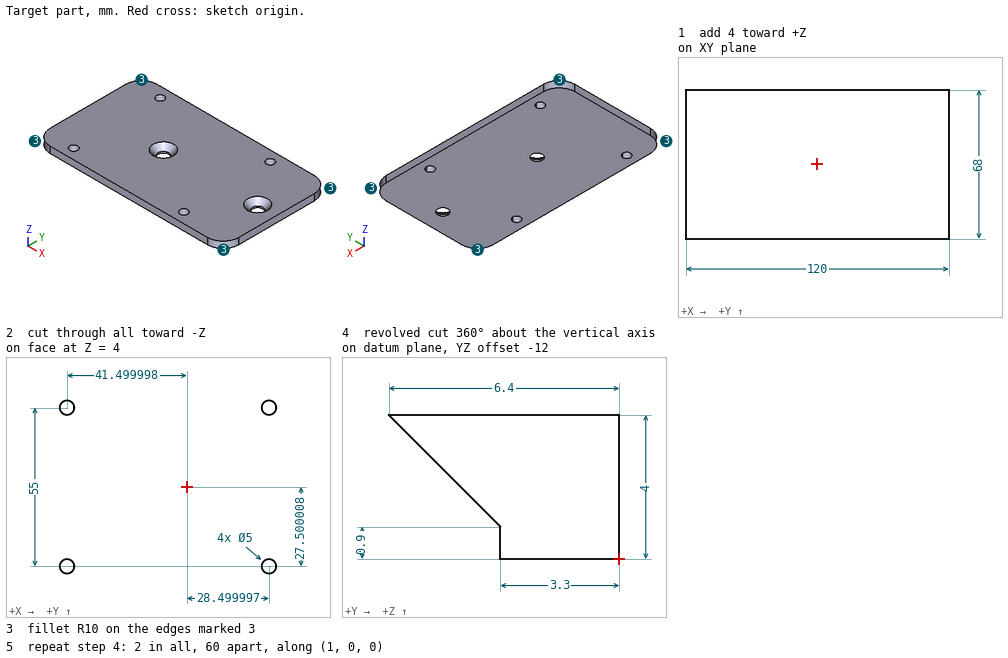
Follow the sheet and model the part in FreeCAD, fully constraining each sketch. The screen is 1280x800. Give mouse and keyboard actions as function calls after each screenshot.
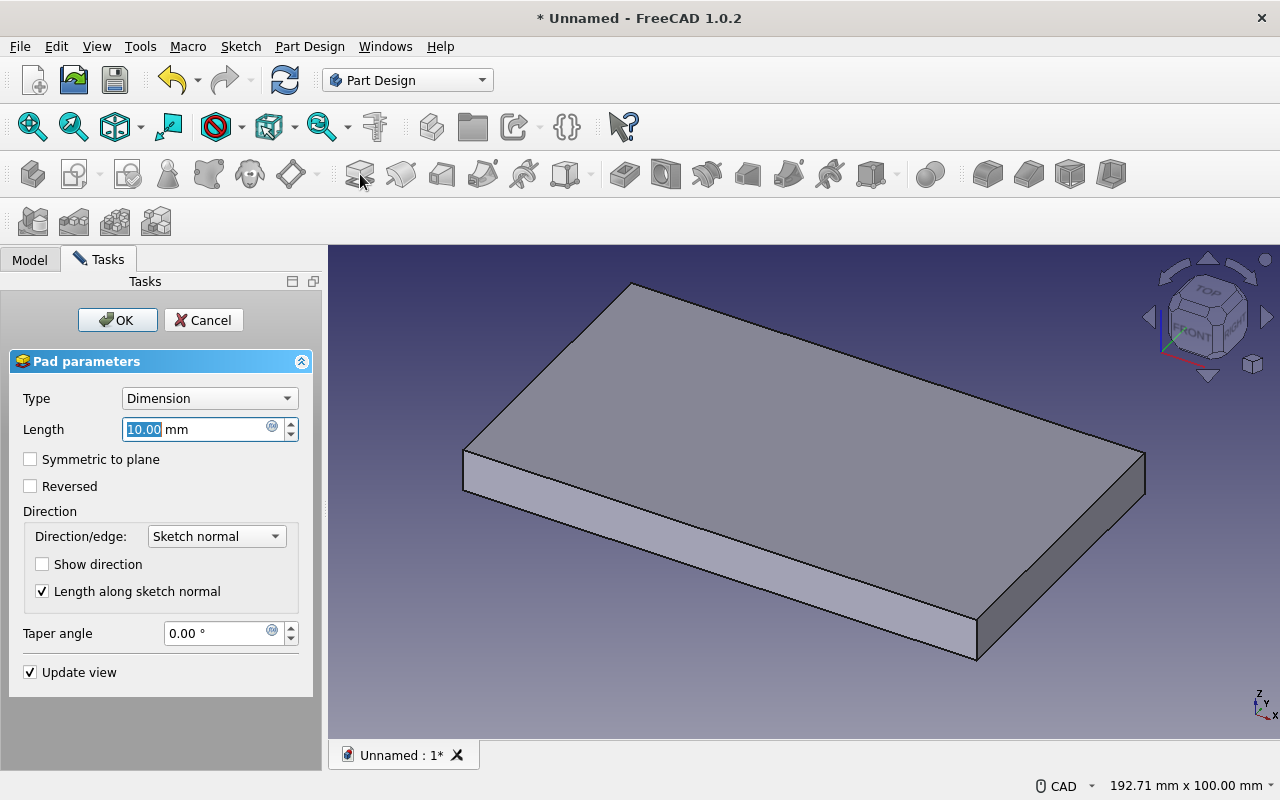
text(4)
key(Tab)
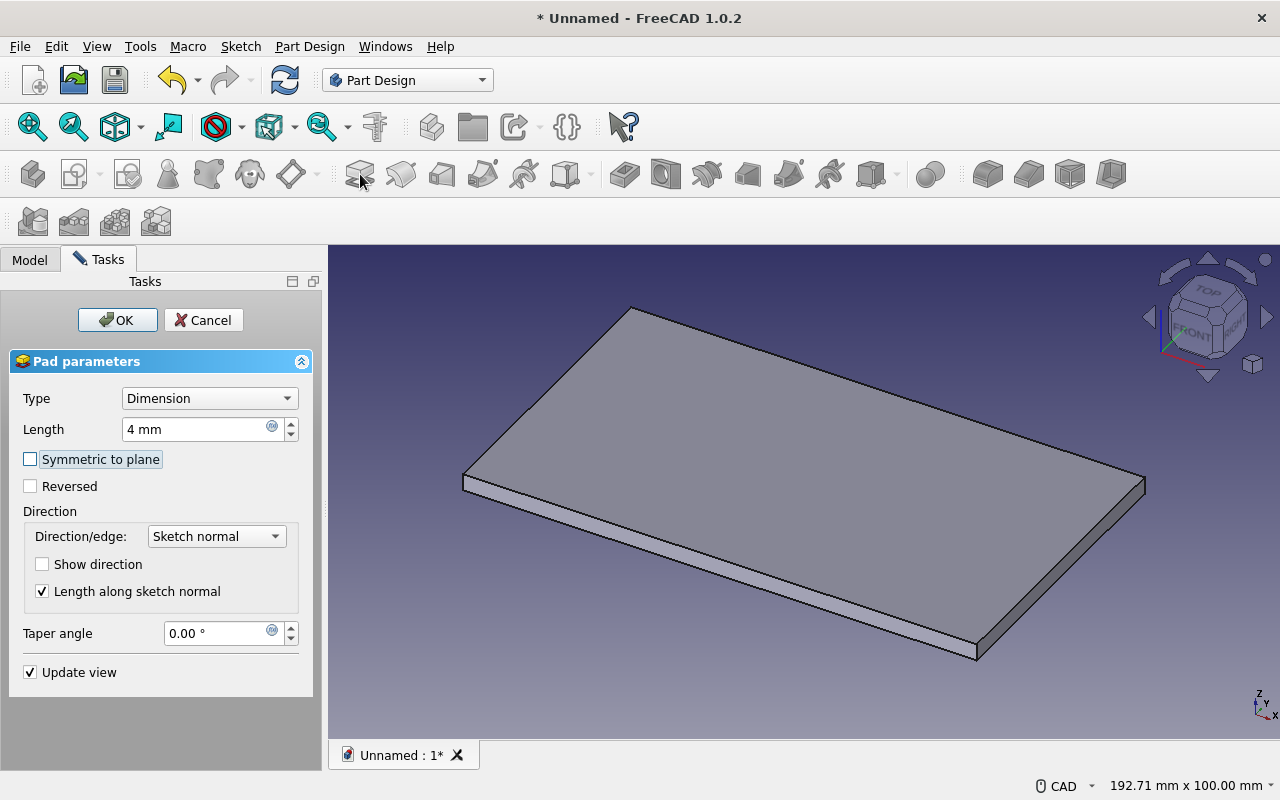
click(118, 320)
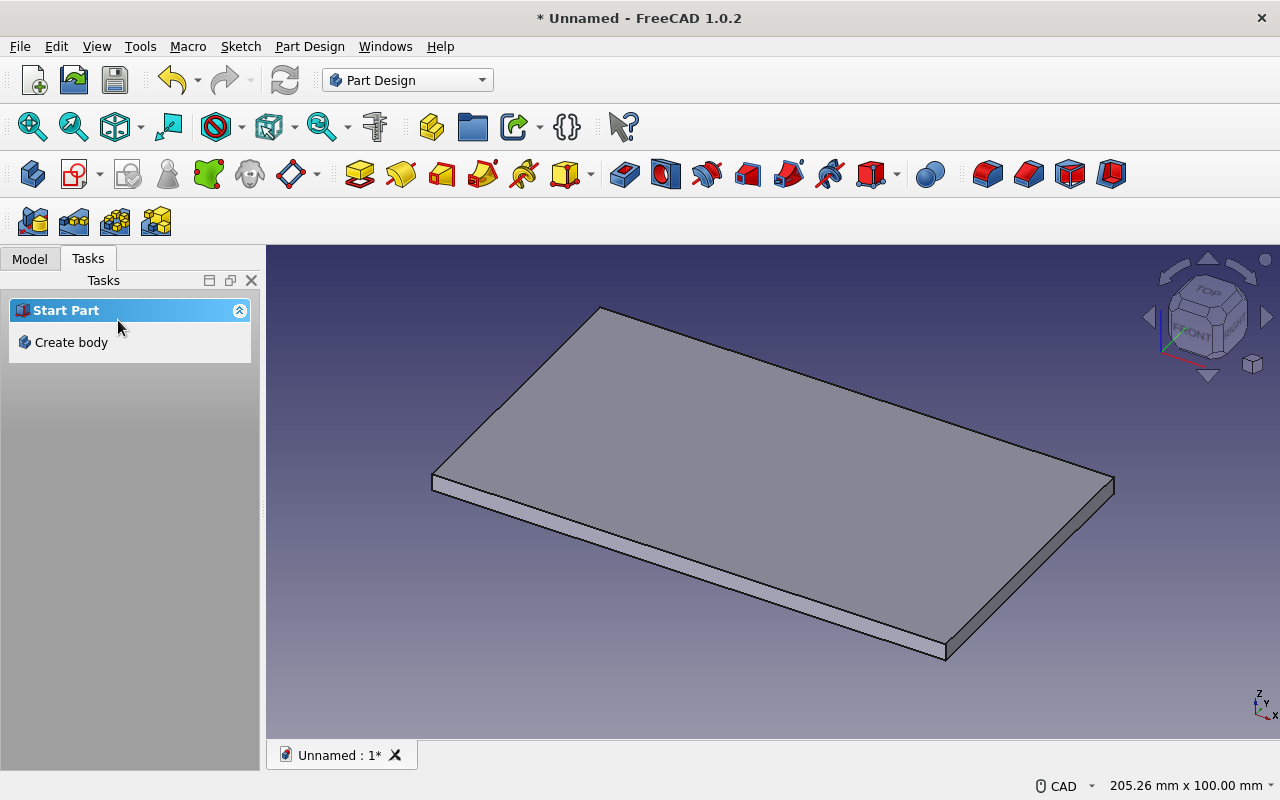
click(846, 499)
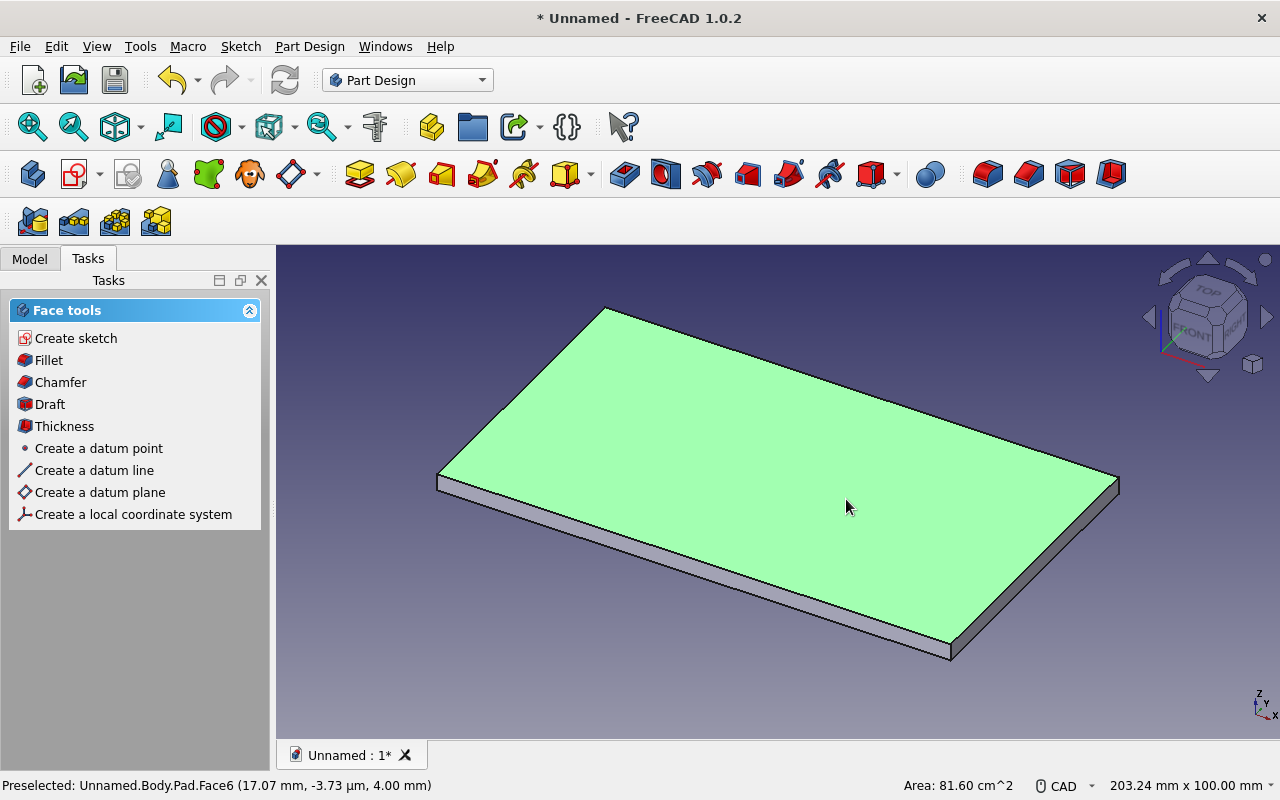
click(74, 174)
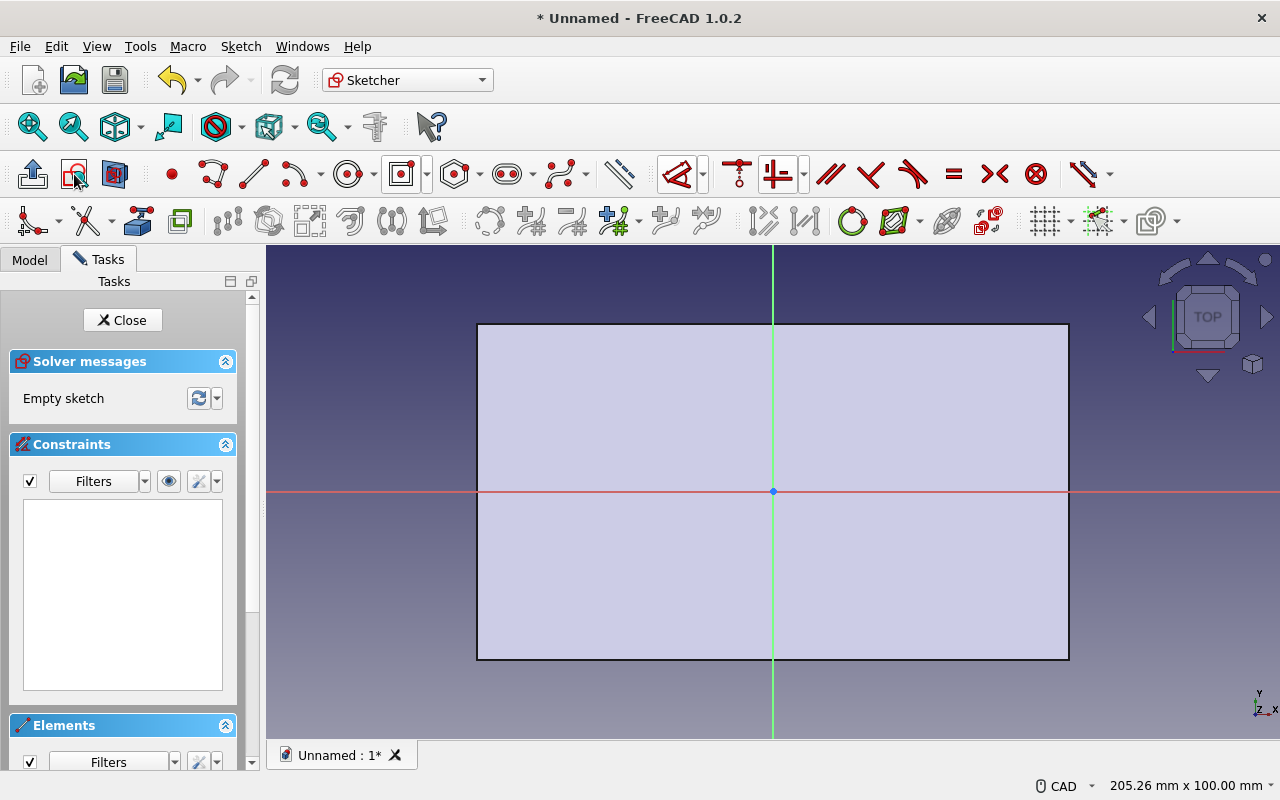
click(348, 174)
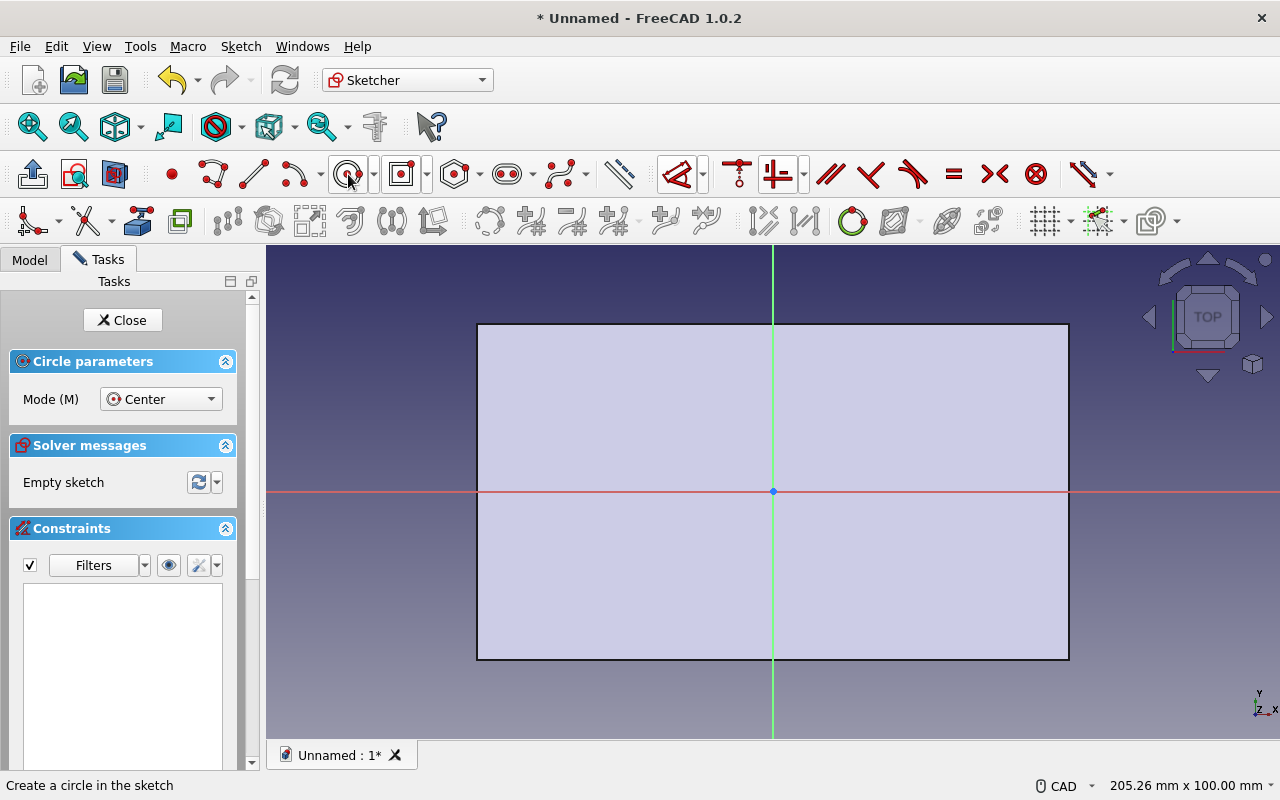
scroll(914, 628, up, 4)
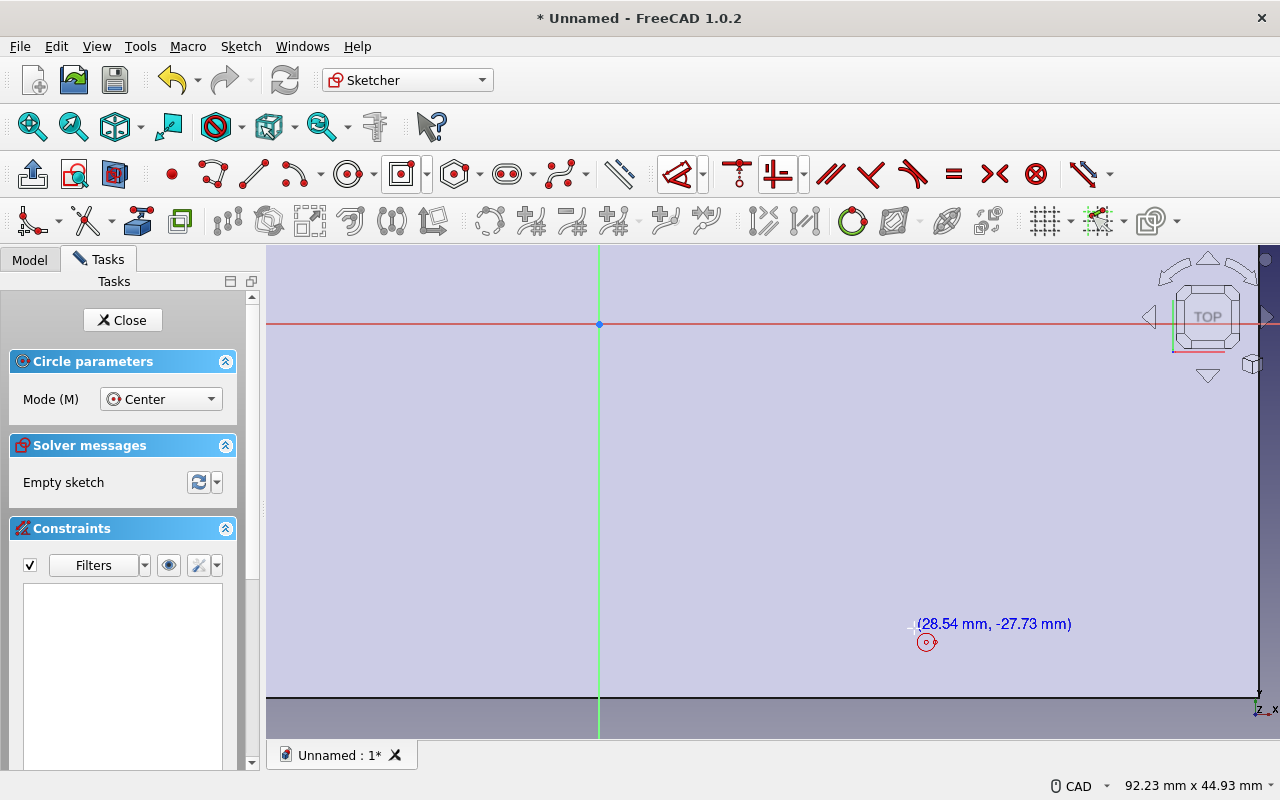
click(913, 627)
move(932, 607)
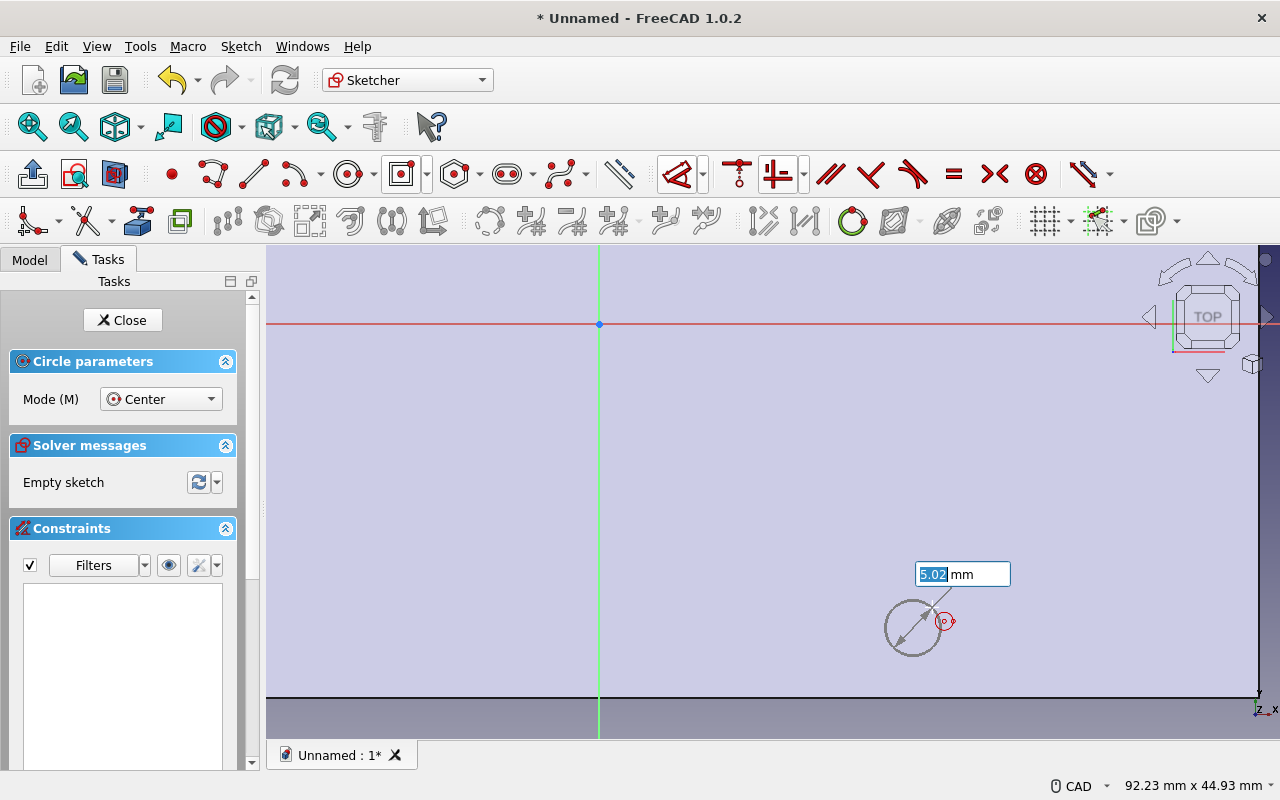
text(5)
key(Return)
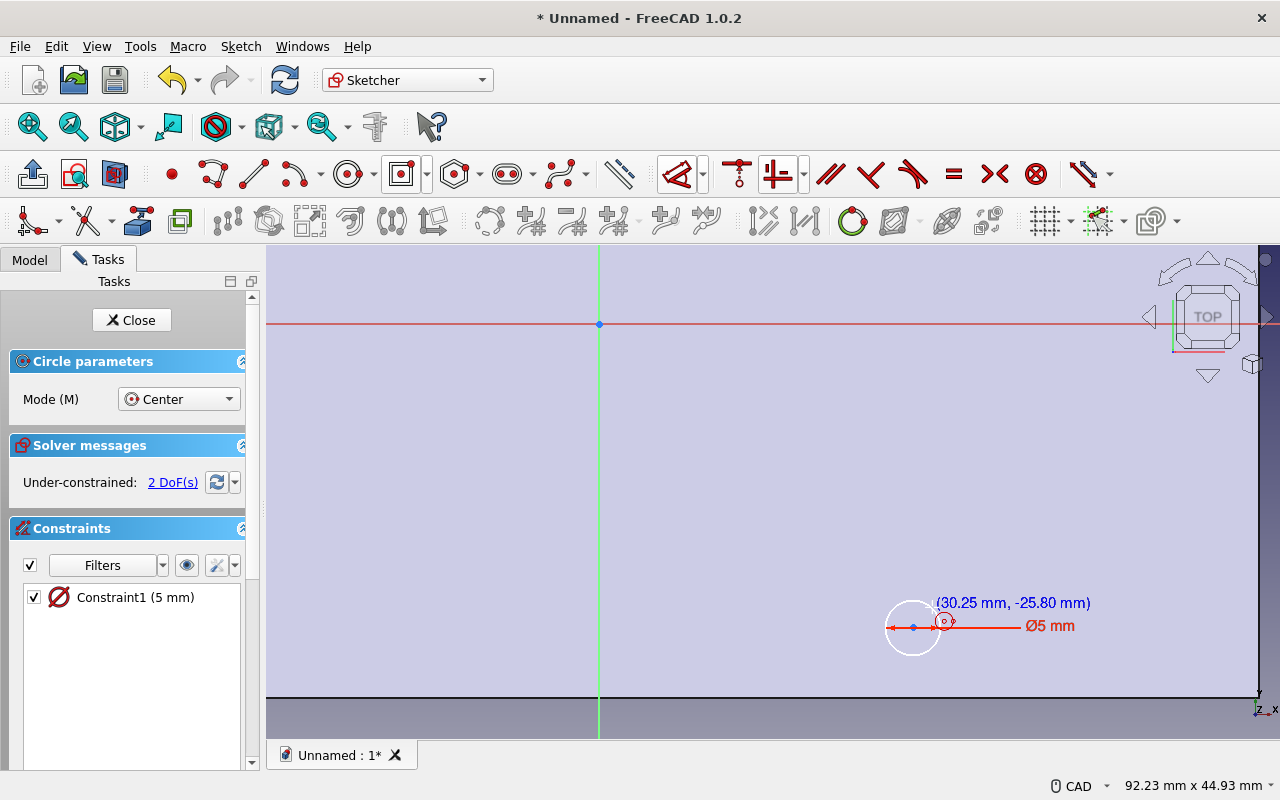
scroll(849, 629, down, 4)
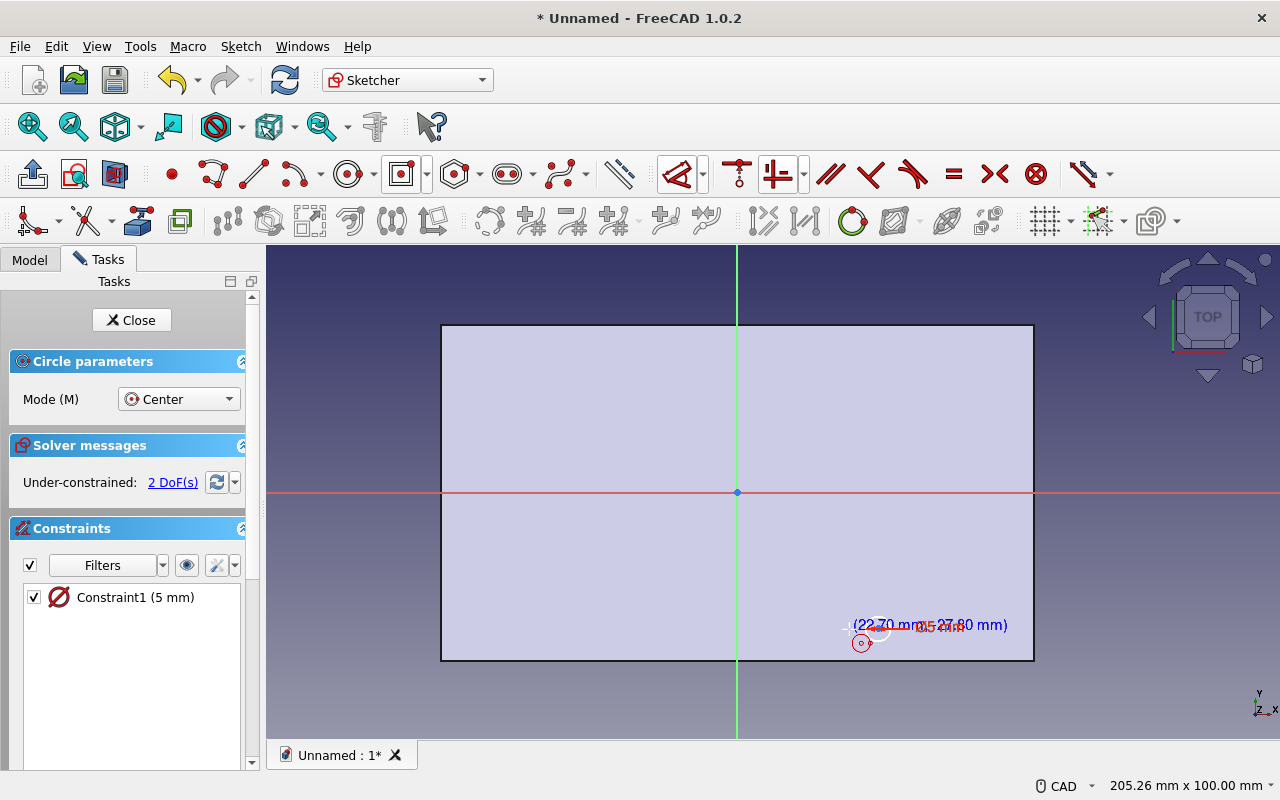
scroll(532, 357, up, 4)